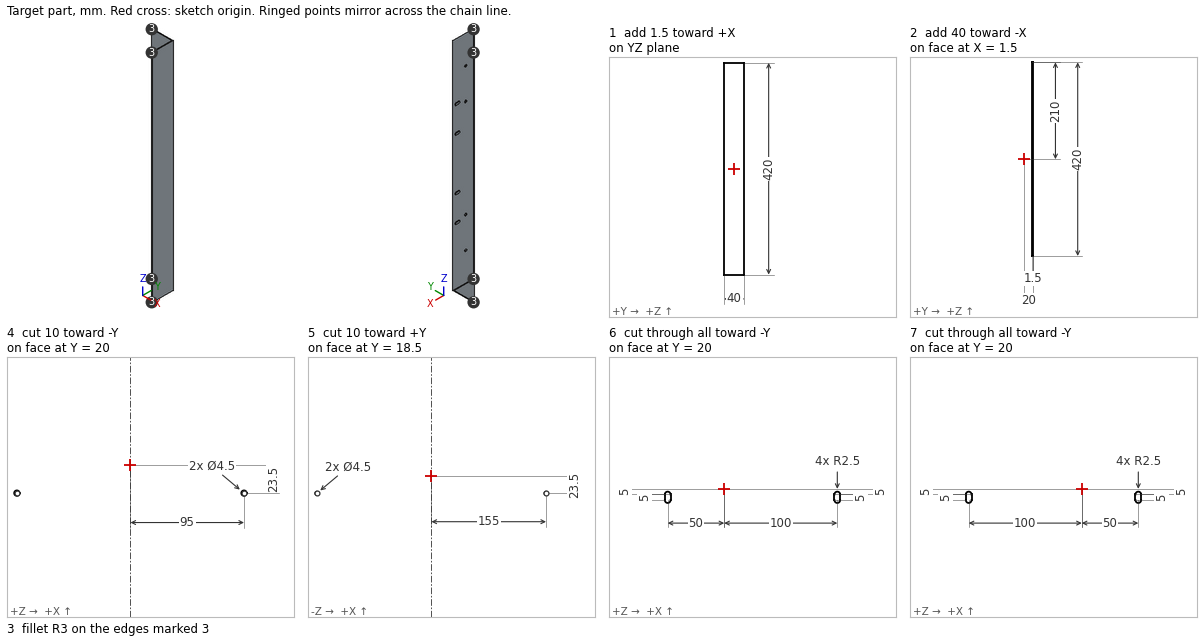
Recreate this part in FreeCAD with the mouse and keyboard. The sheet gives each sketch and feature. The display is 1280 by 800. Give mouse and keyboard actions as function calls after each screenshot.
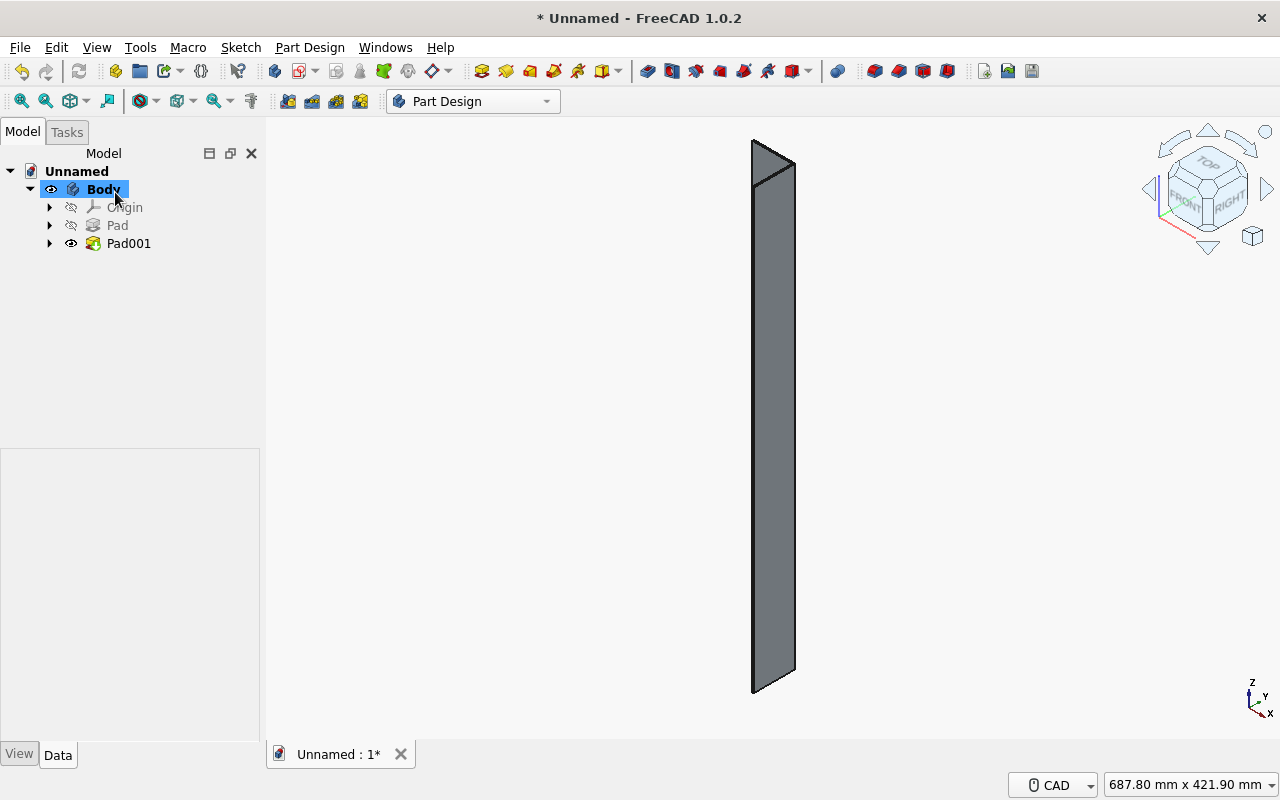
key(2)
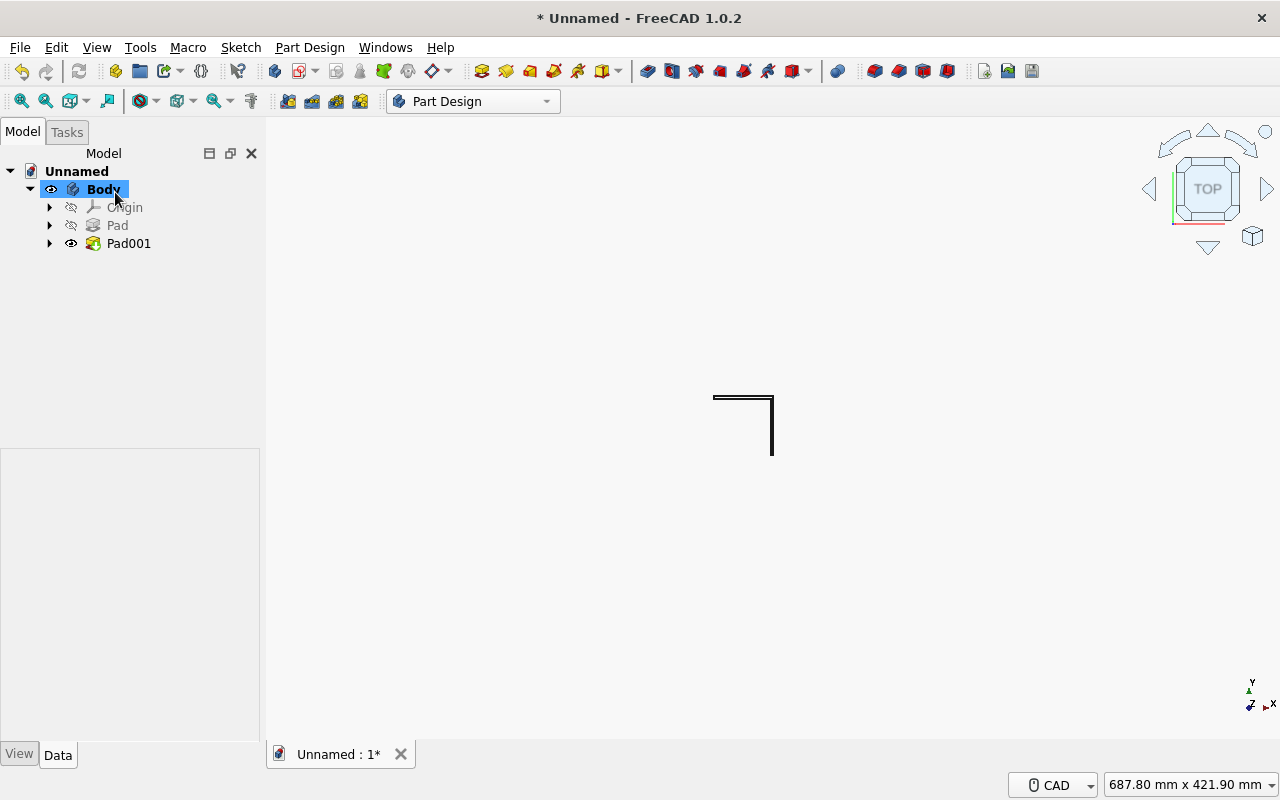
click(22, 102)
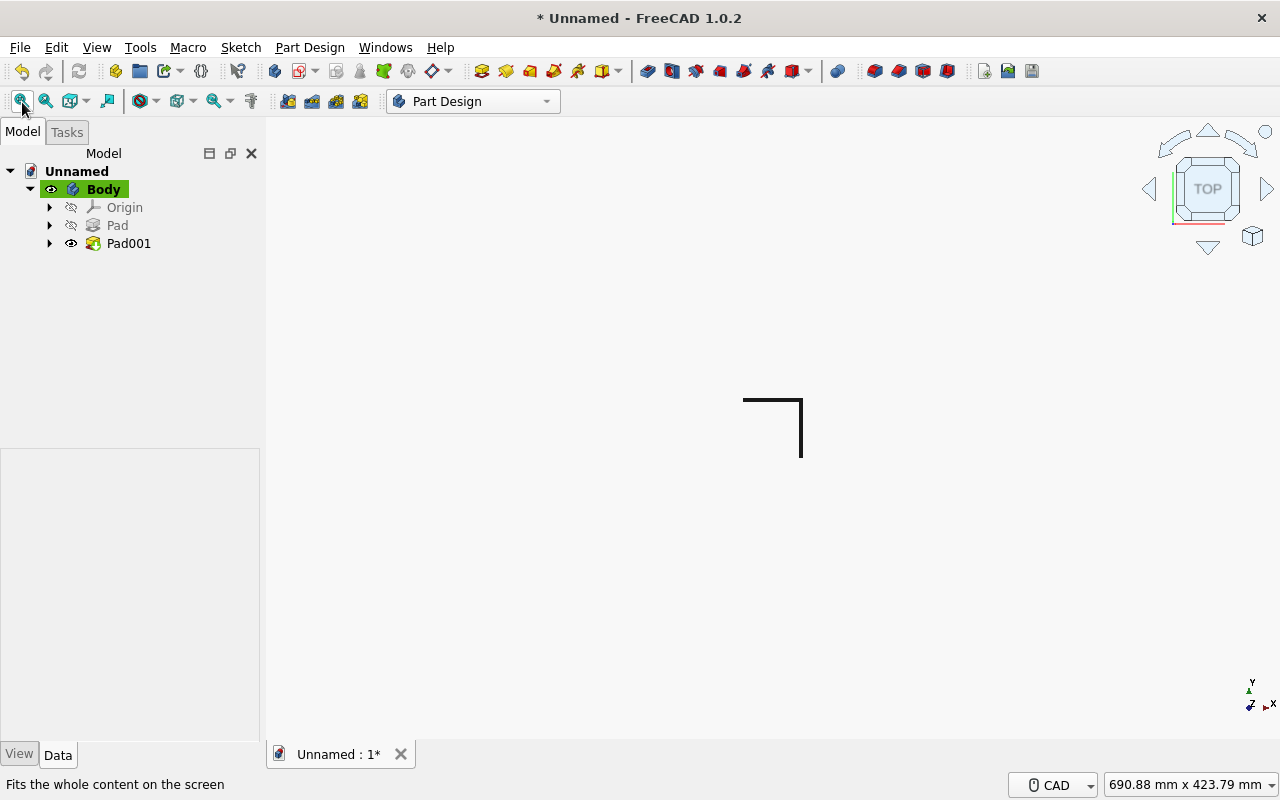
scroll(744, 399, up, 15)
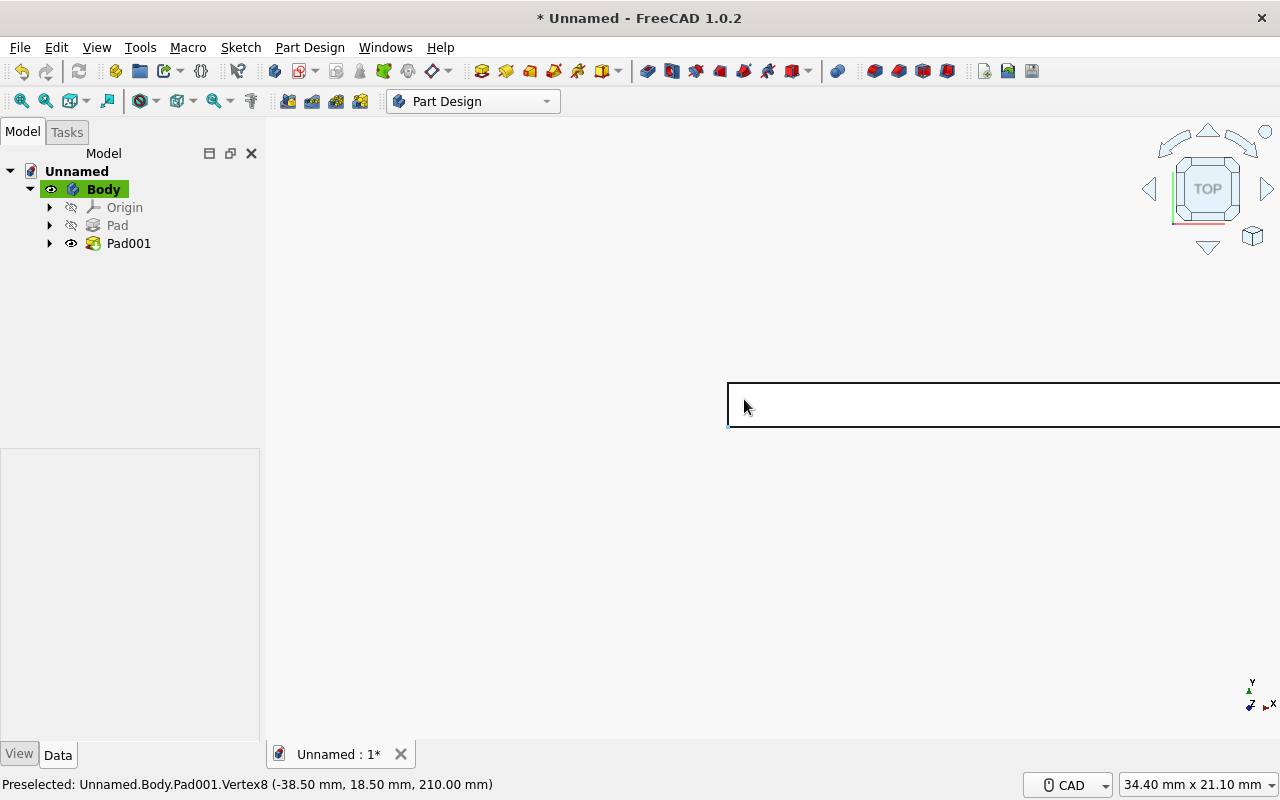
click(728, 404)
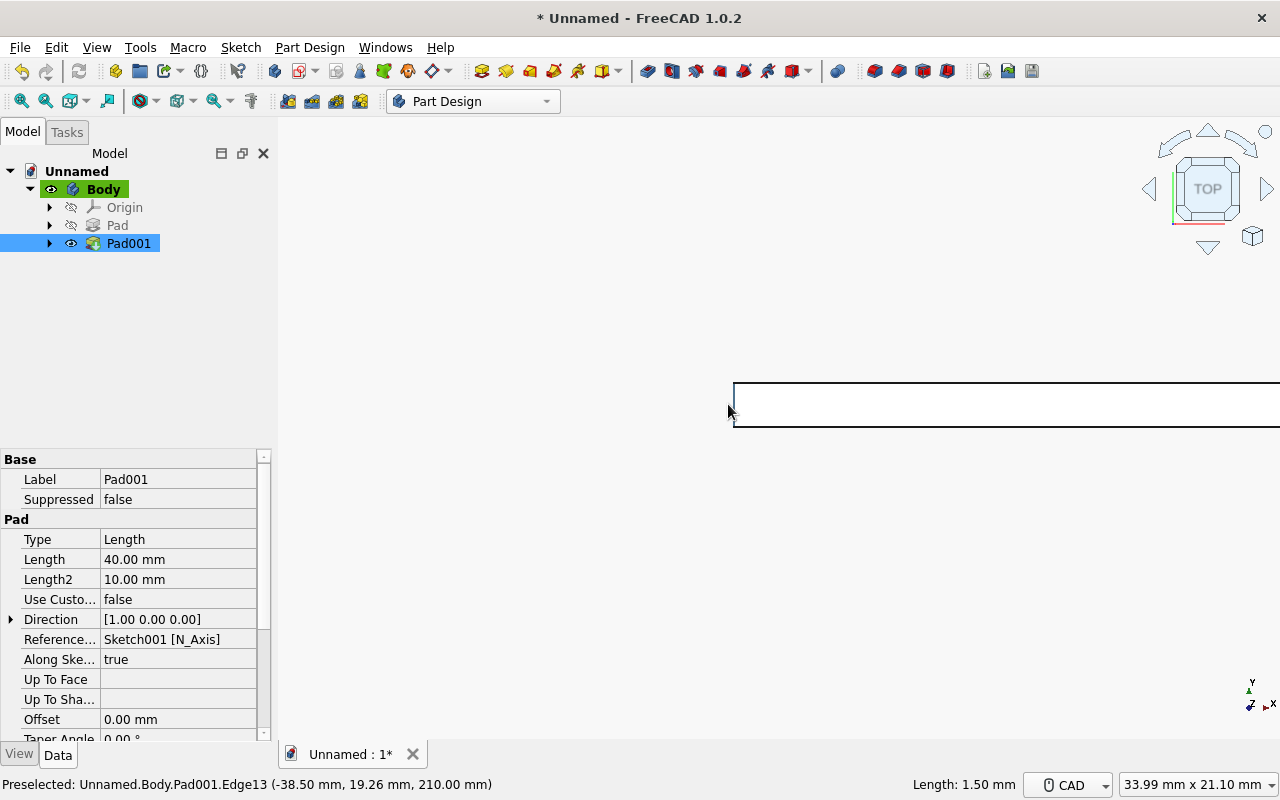
click(22, 102)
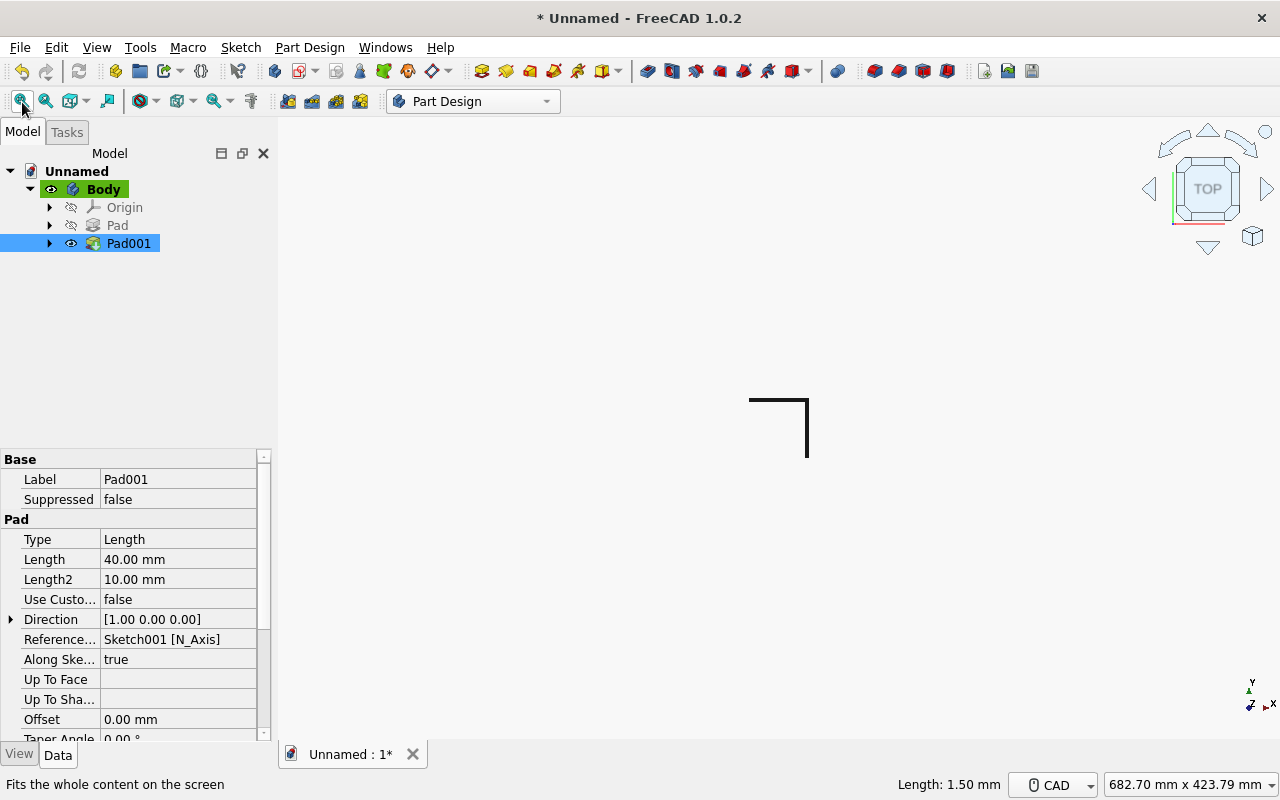
key(1)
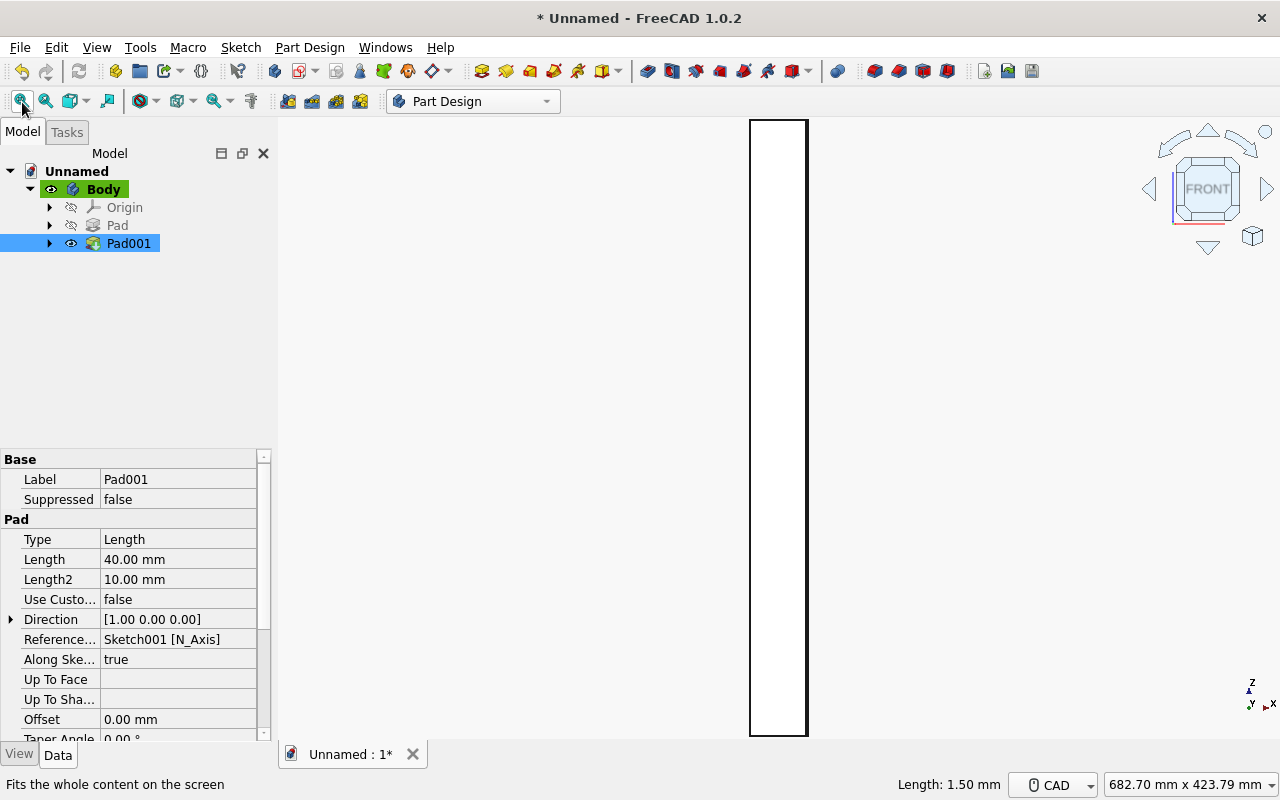
key(3)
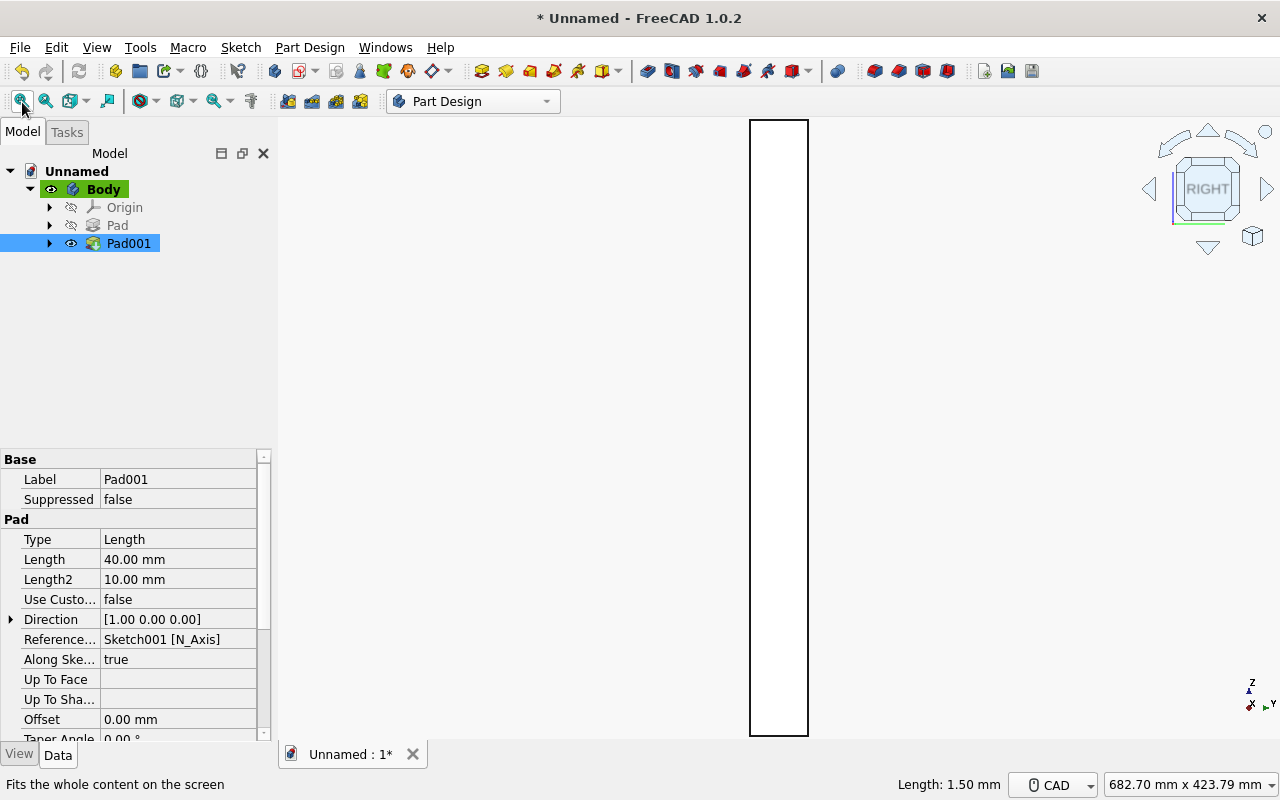
key(5)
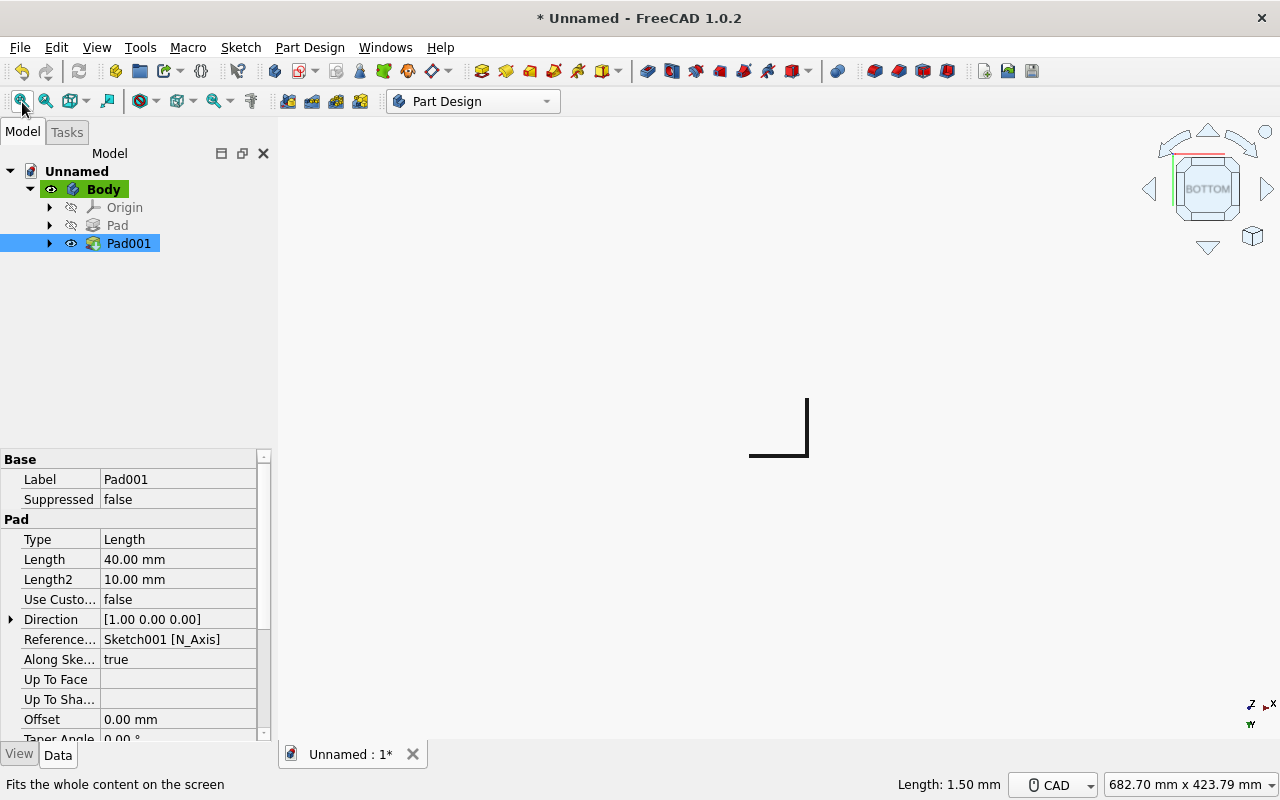
click(22, 102)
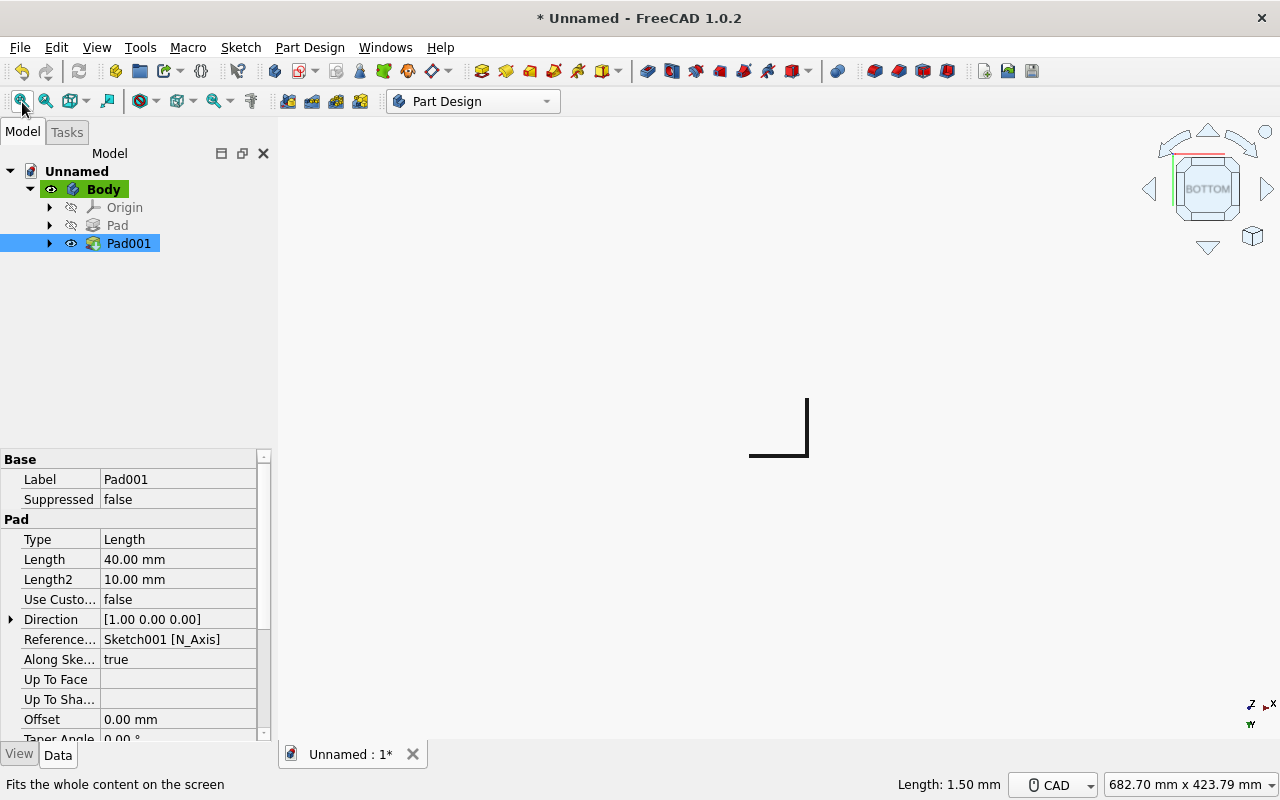
scroll(750, 455, up, 15)